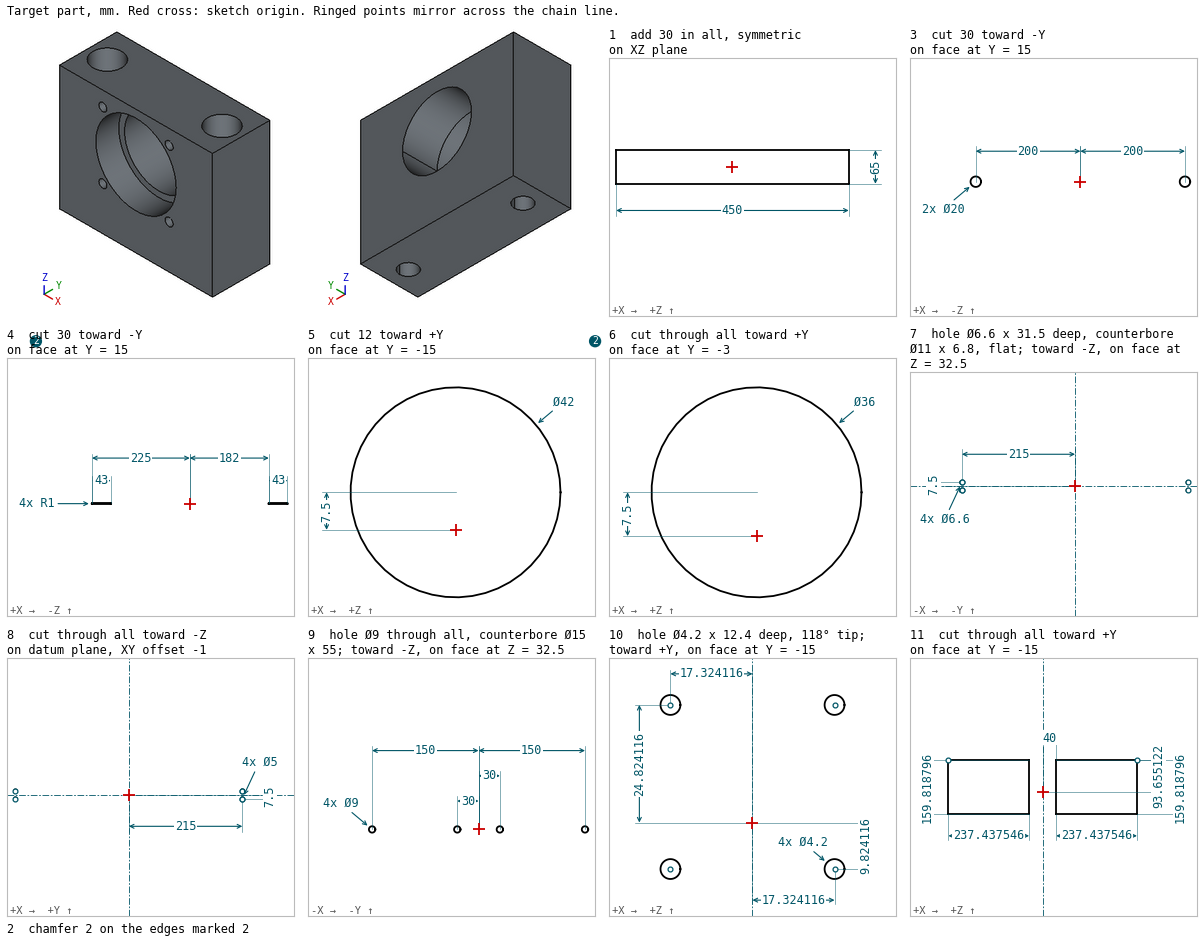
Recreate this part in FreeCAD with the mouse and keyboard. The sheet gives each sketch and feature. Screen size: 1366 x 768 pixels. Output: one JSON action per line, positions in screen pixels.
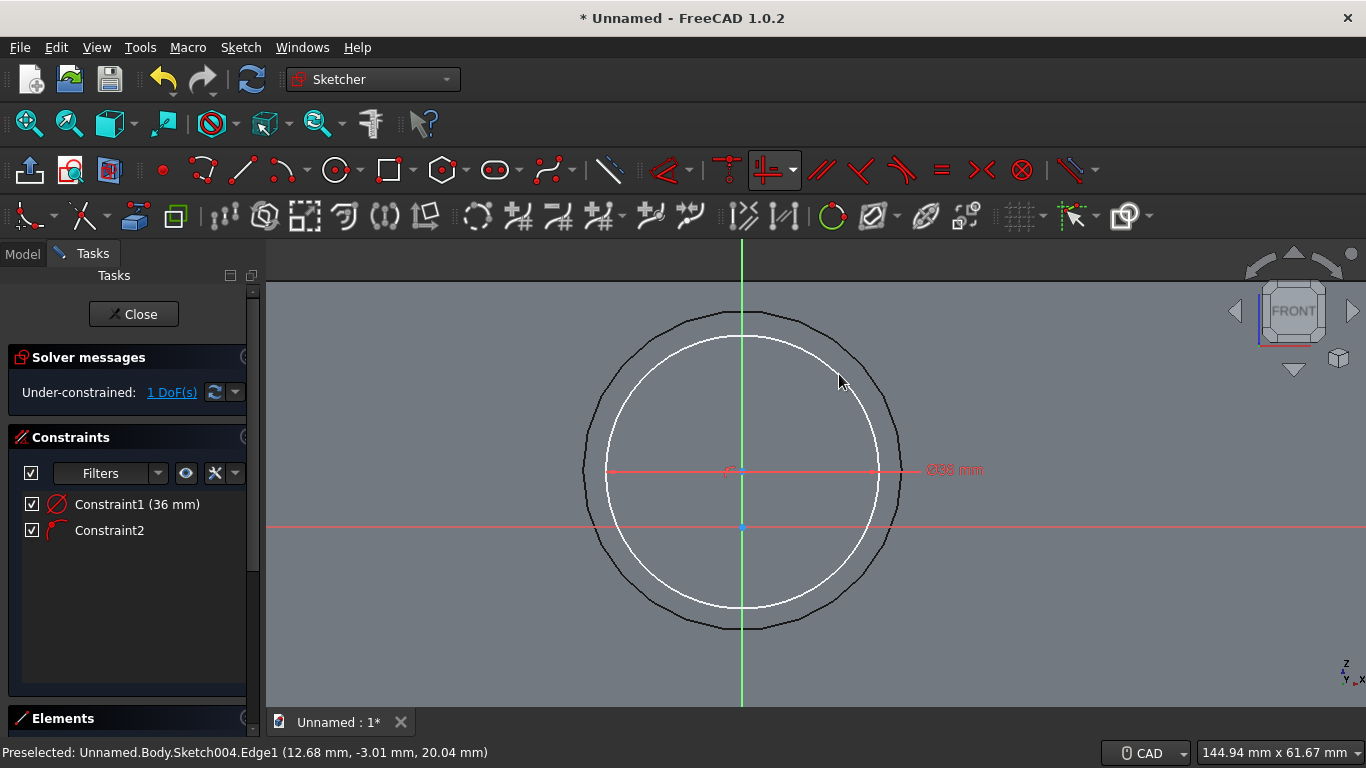
{"action": "key", "text": "d"}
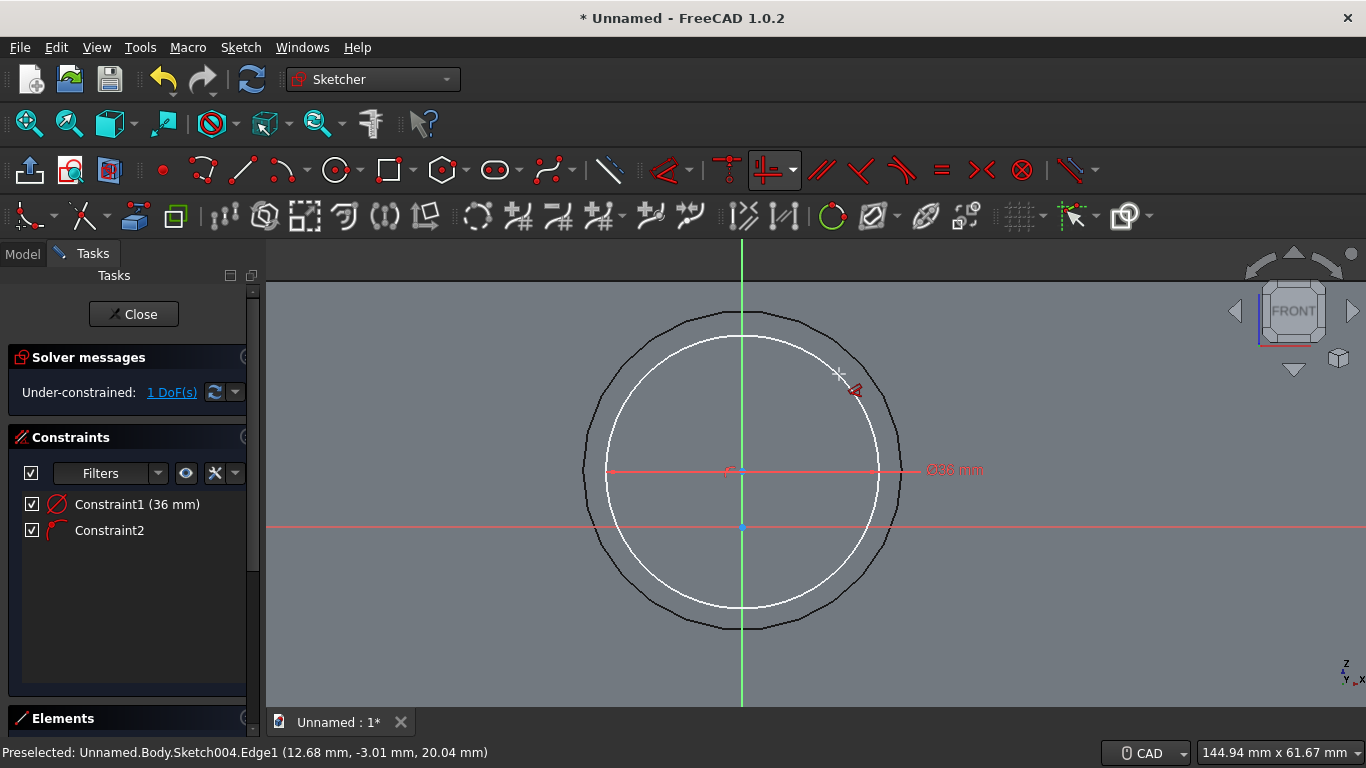
{"action": "left_click", "coordinate": [742, 472]}
{"action": "left_click", "coordinate": [776, 500]}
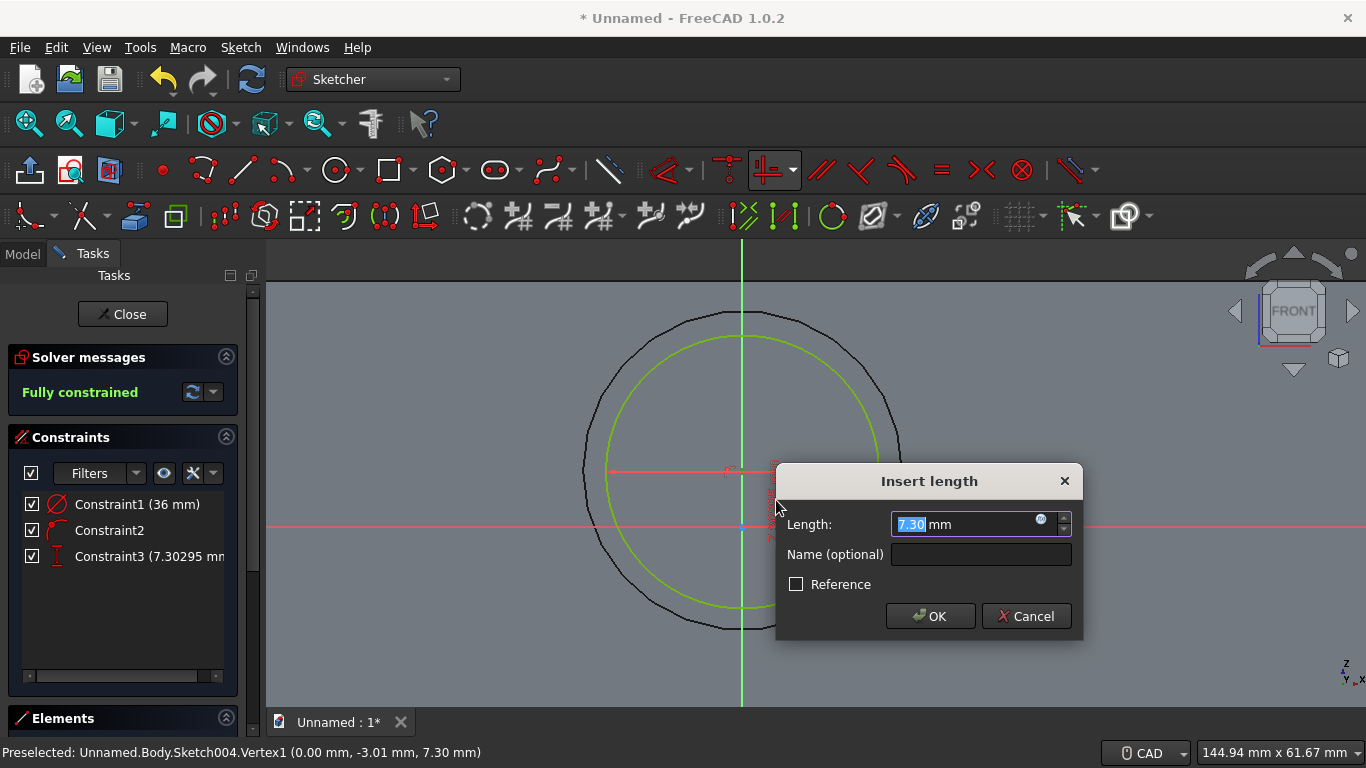
{"action": "type", "text": "7.5"}
{"action": "key", "text": "Return"}
{"action": "key", "text": "Escape"}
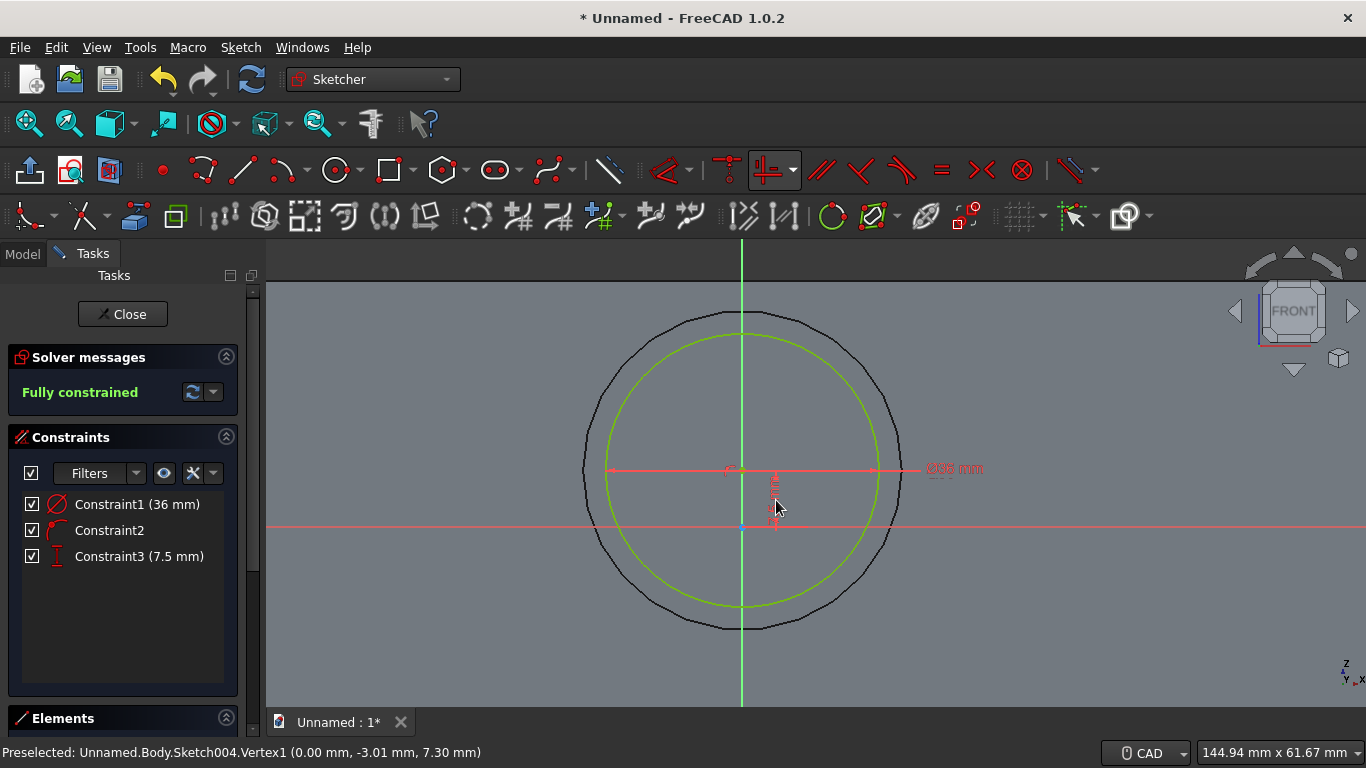
{"action": "left_click", "coordinate": [123, 314]}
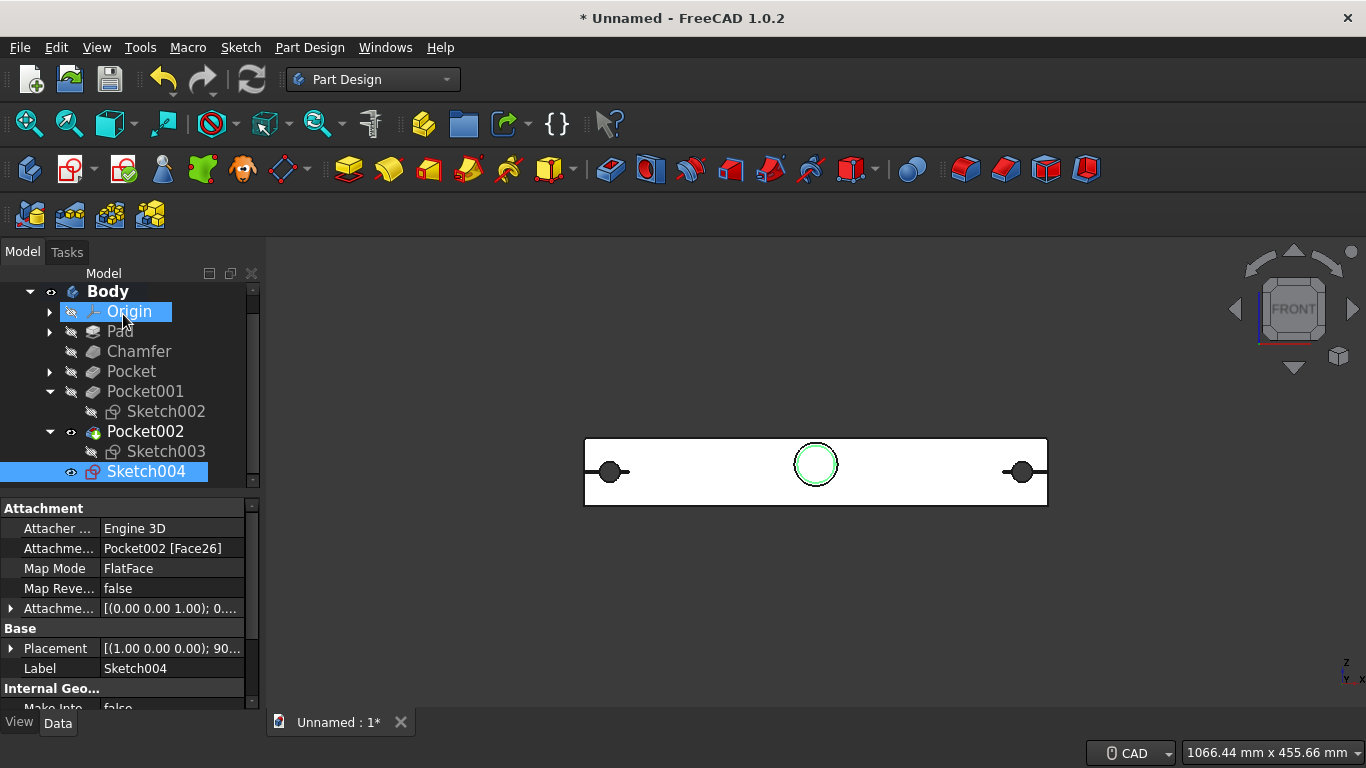
{"action": "left_click", "coordinate": [612, 170]}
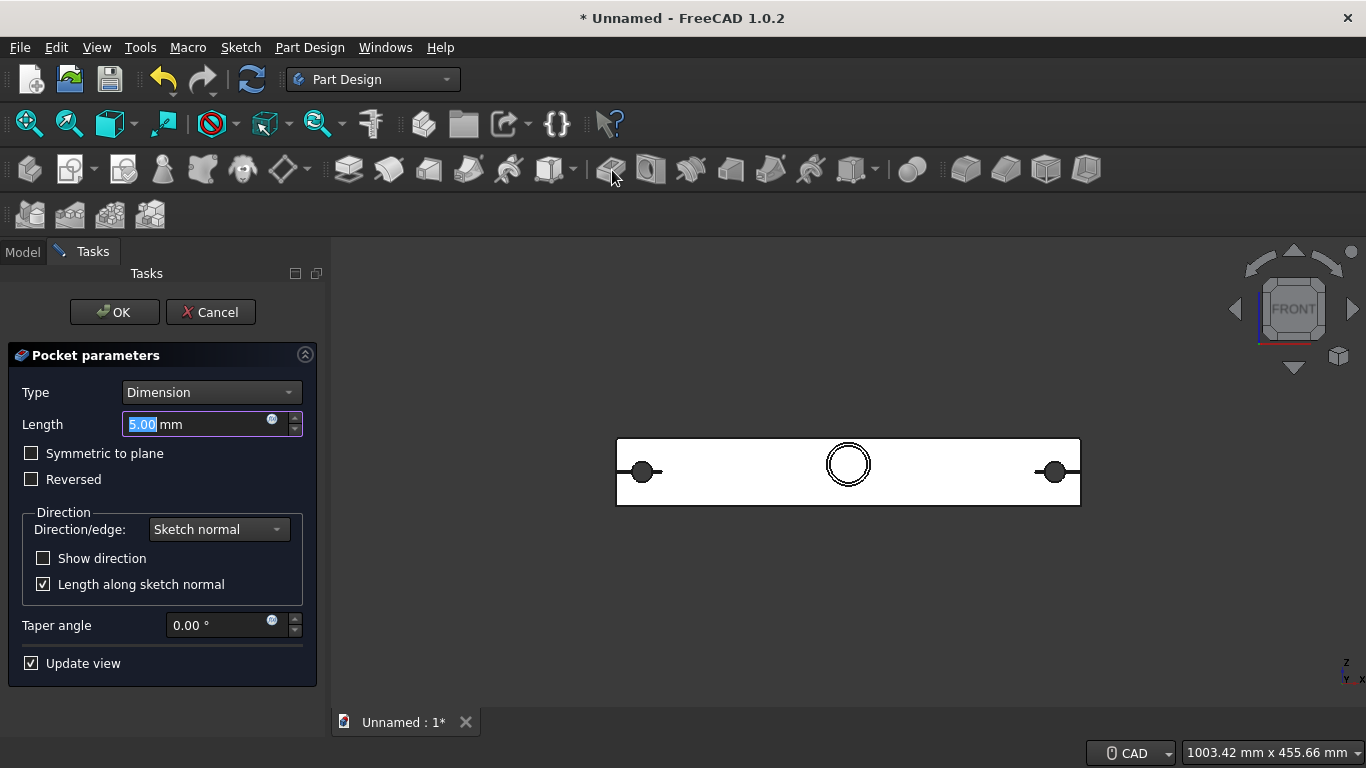
{"action": "left_click", "coordinate": [212, 392]}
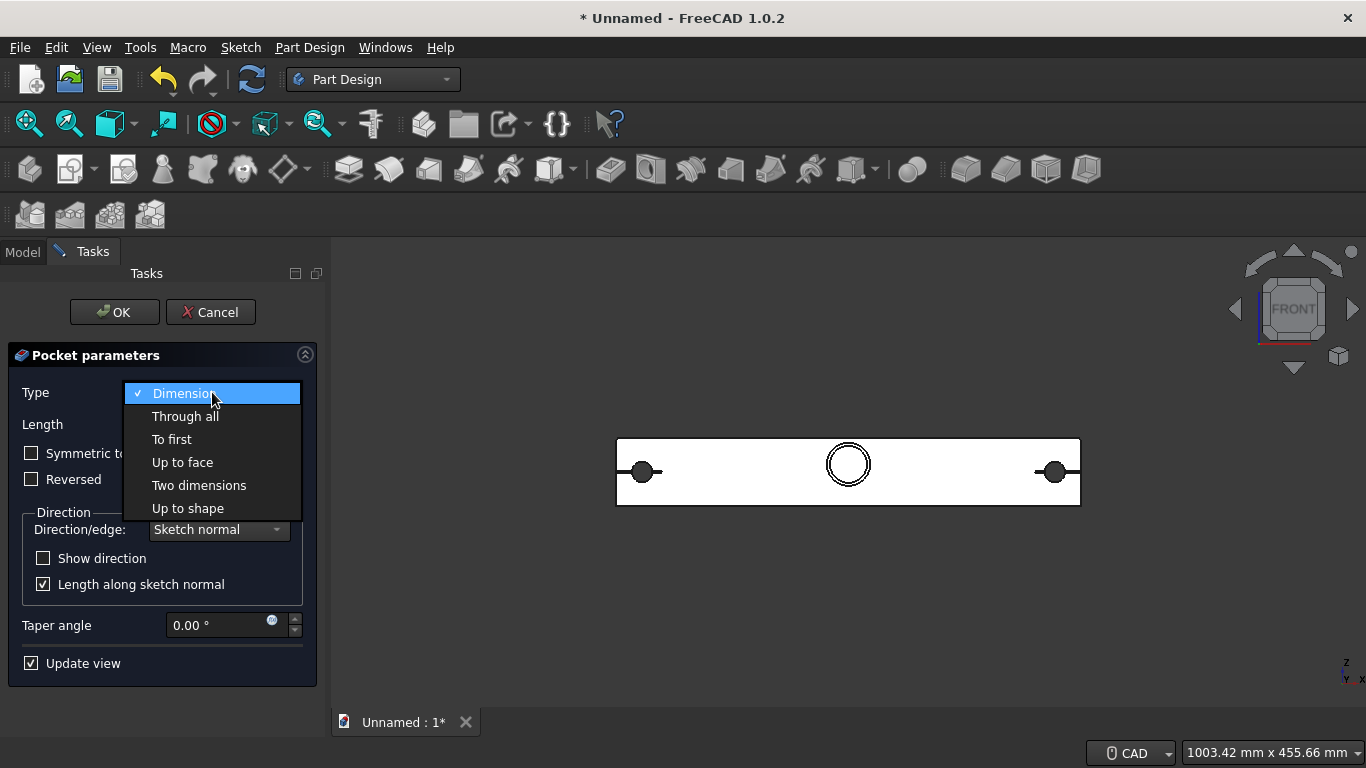
{"action": "left_click", "coordinate": [212, 416]}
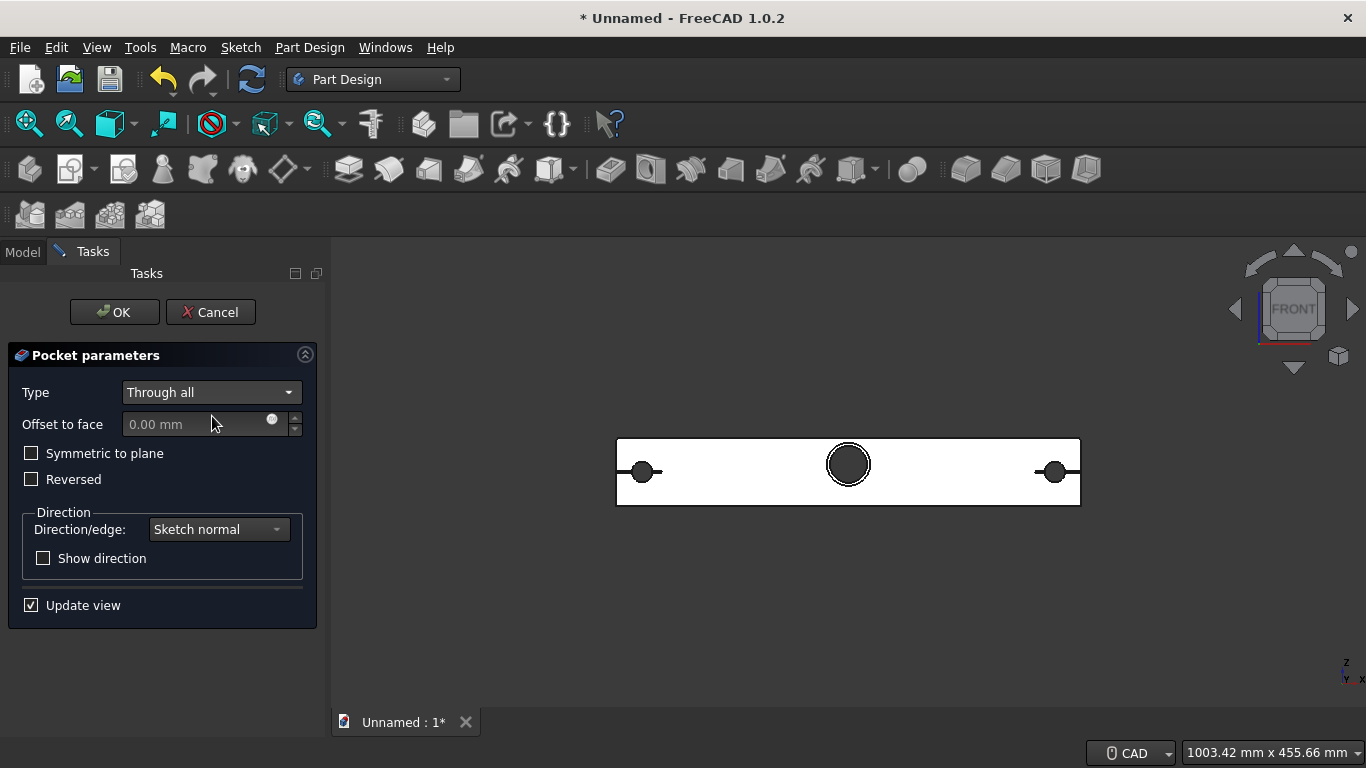
{"action": "left_click", "coordinate": [115, 312]}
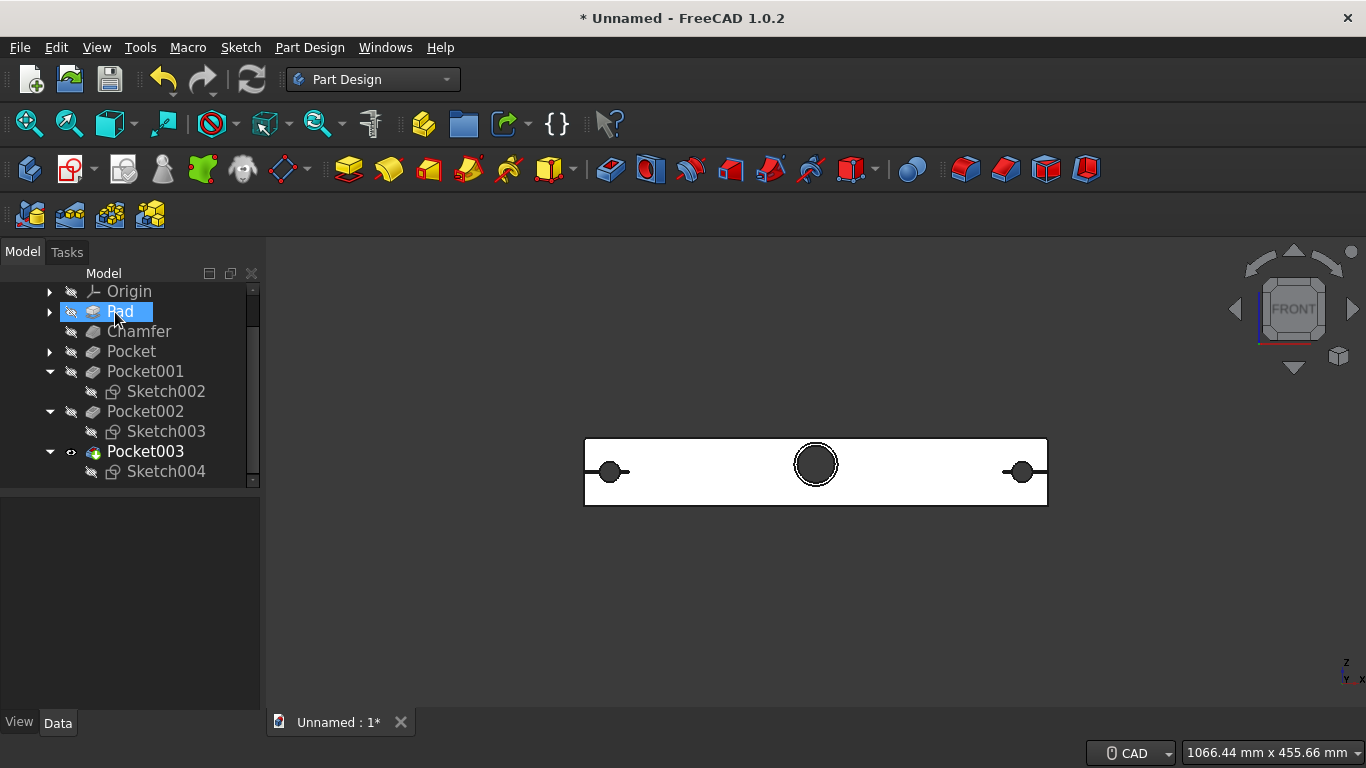
{"action": "key", "text": "v f"}